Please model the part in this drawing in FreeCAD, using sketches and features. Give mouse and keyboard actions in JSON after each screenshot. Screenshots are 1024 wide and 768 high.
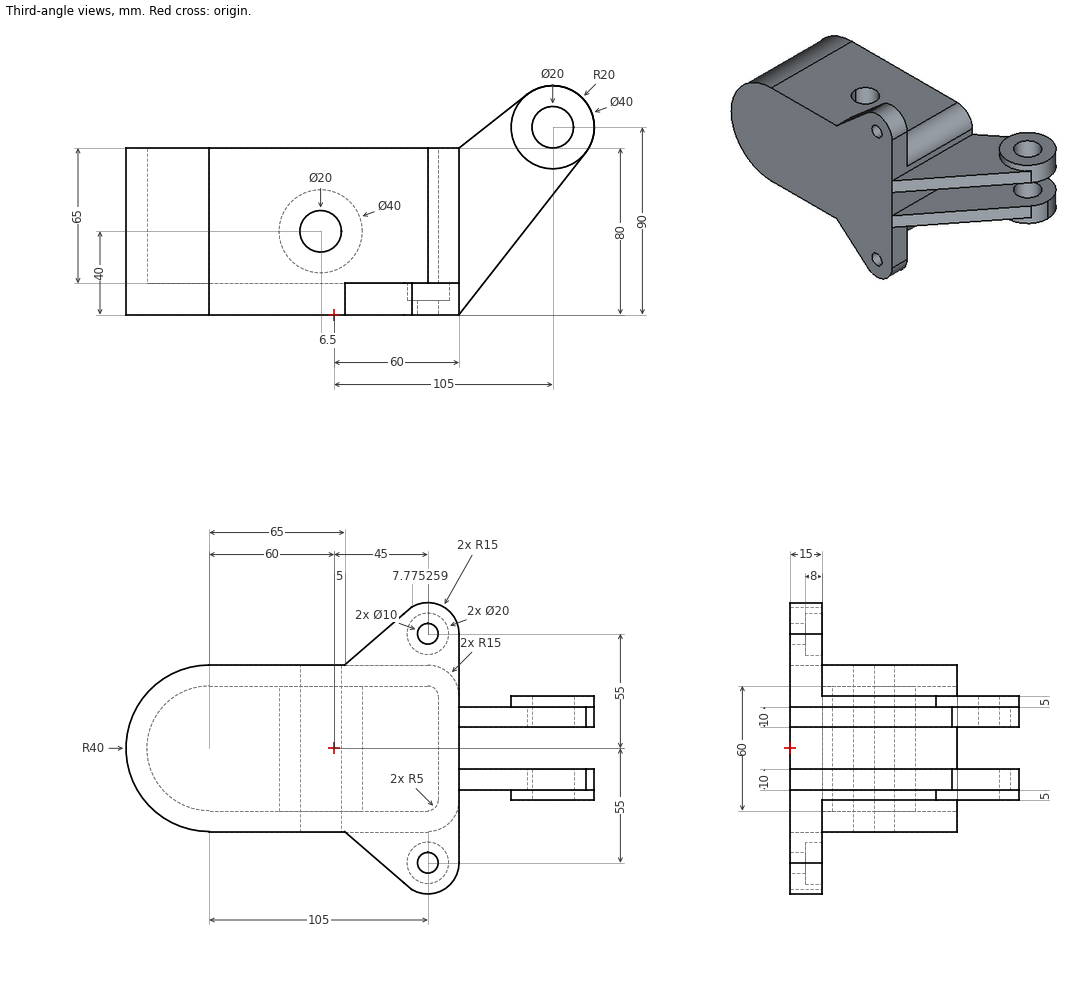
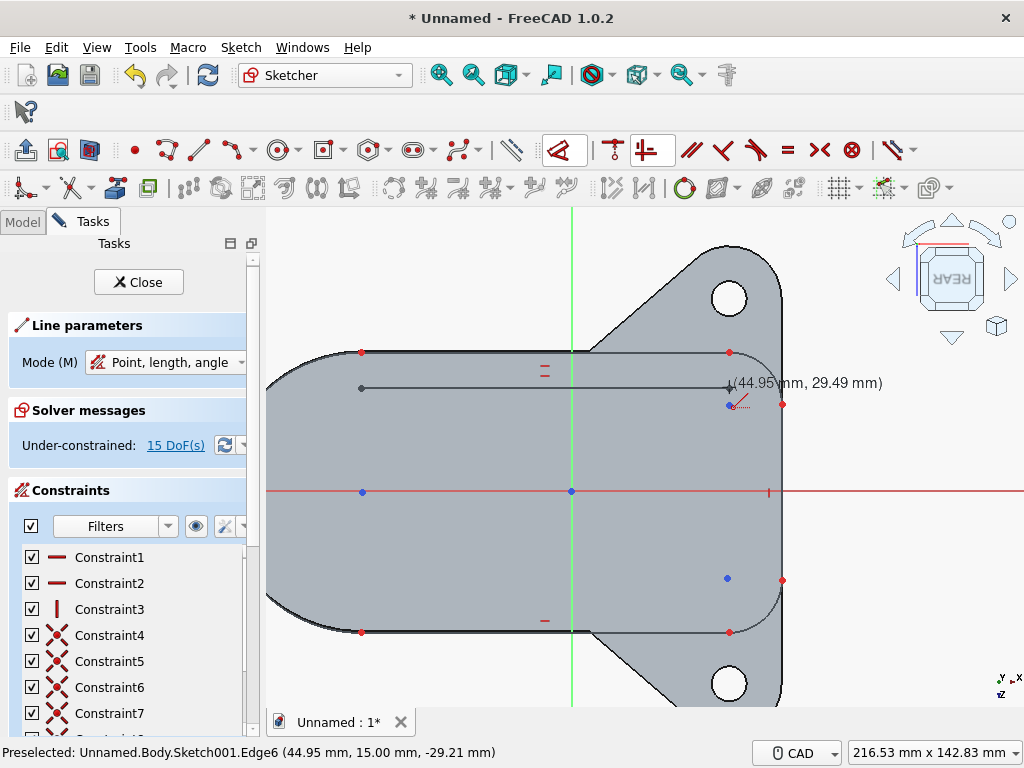
{"action": "left_click", "coordinate": [747, 404]}
{"action": "left_click", "coordinate": [747, 579]}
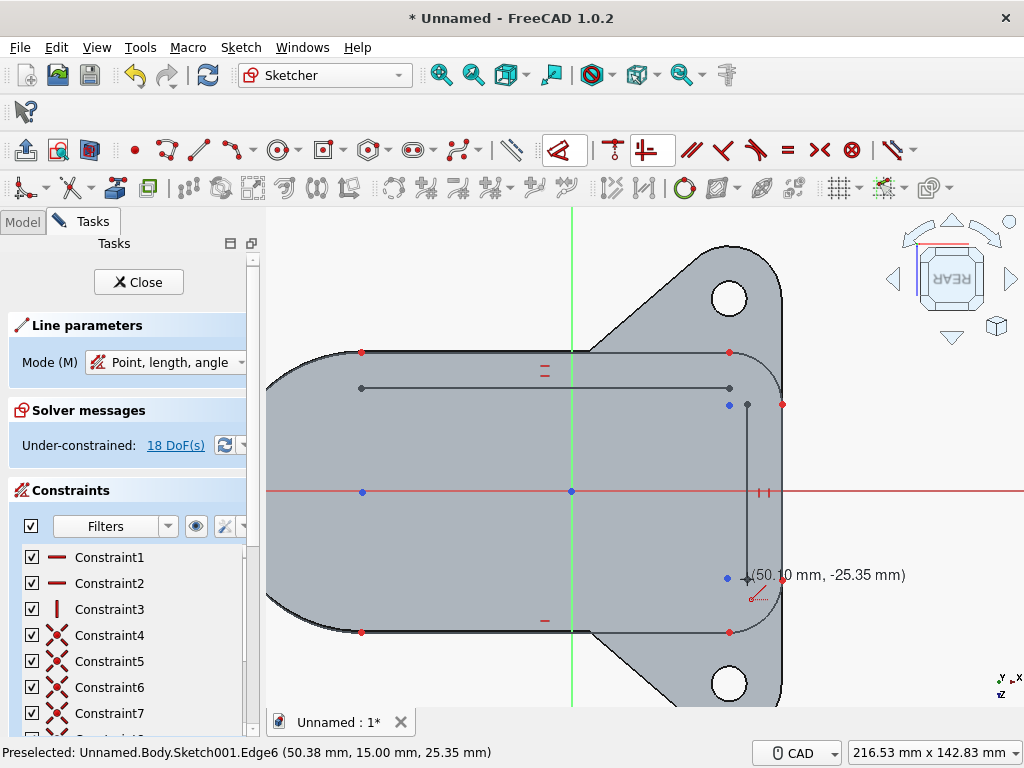
{"action": "left_click", "coordinate": [729, 596]}
{"action": "left_click", "coordinate": [362, 596]}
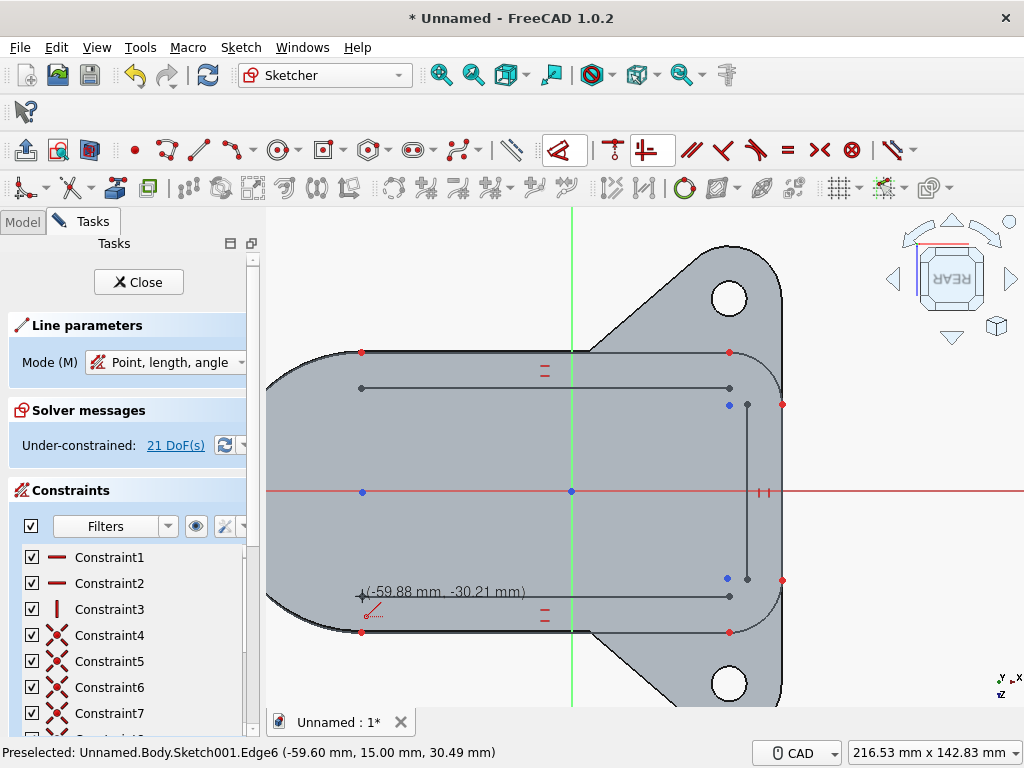
{"action": "left_click", "coordinate": [232, 150]}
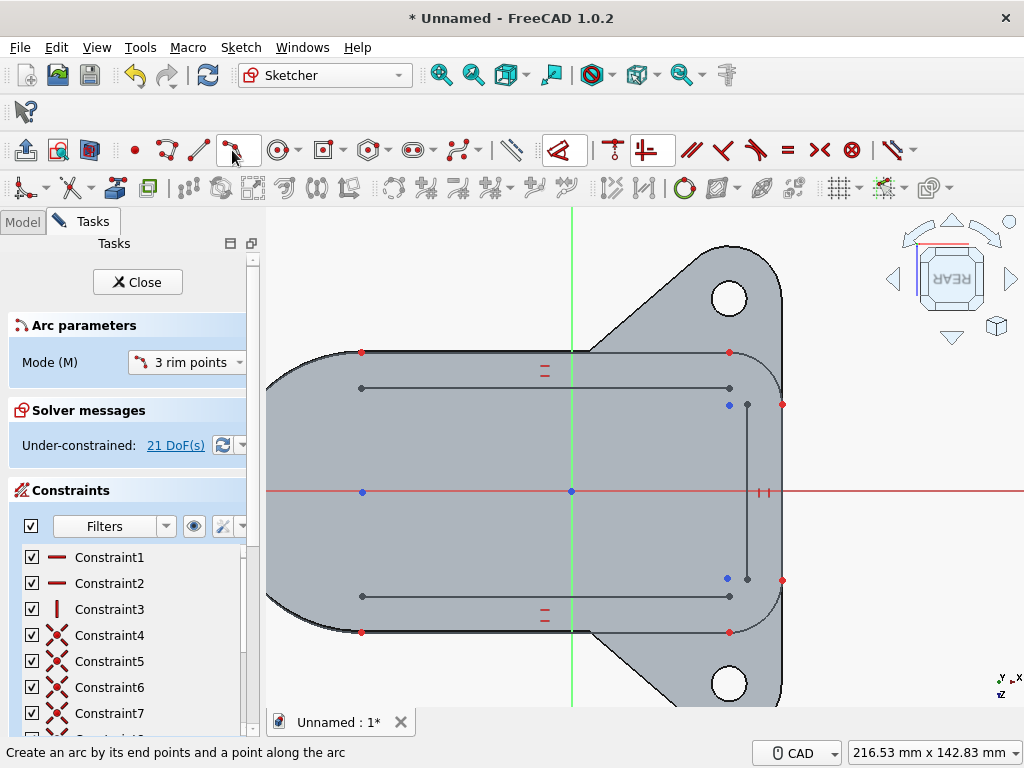
{"action": "left_click", "coordinate": [729, 388]}
{"action": "left_click", "coordinate": [747, 405]}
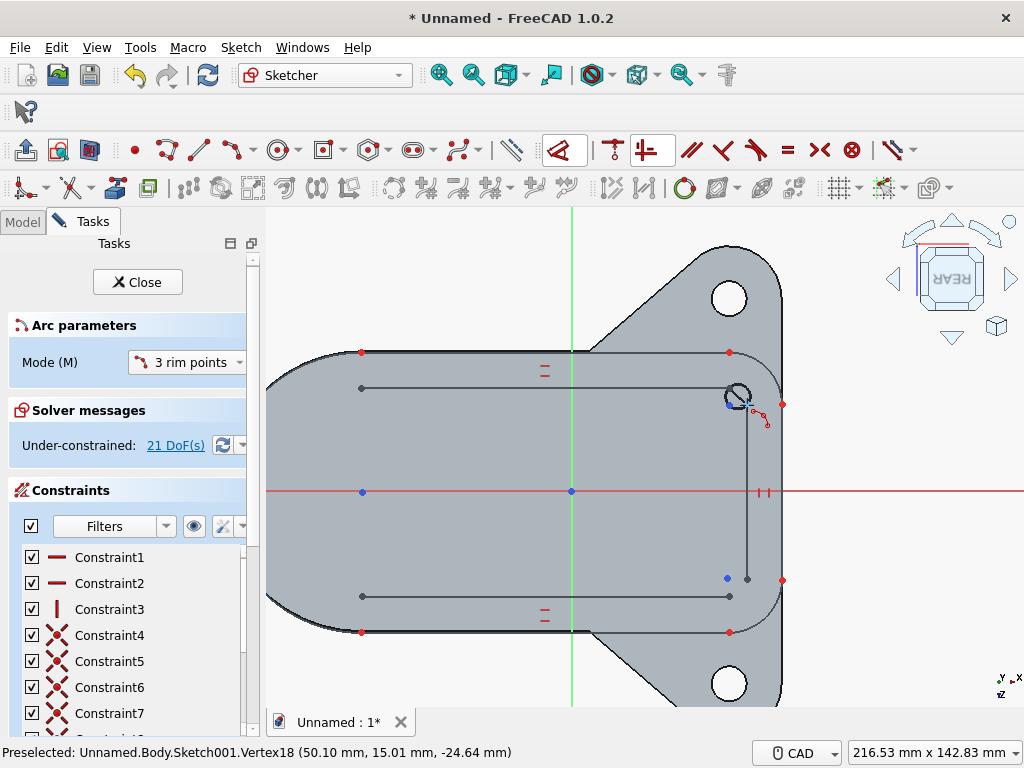
{"action": "scroll", "coordinate": [742, 391], "scroll_direction": "up", "scroll_amount": 6}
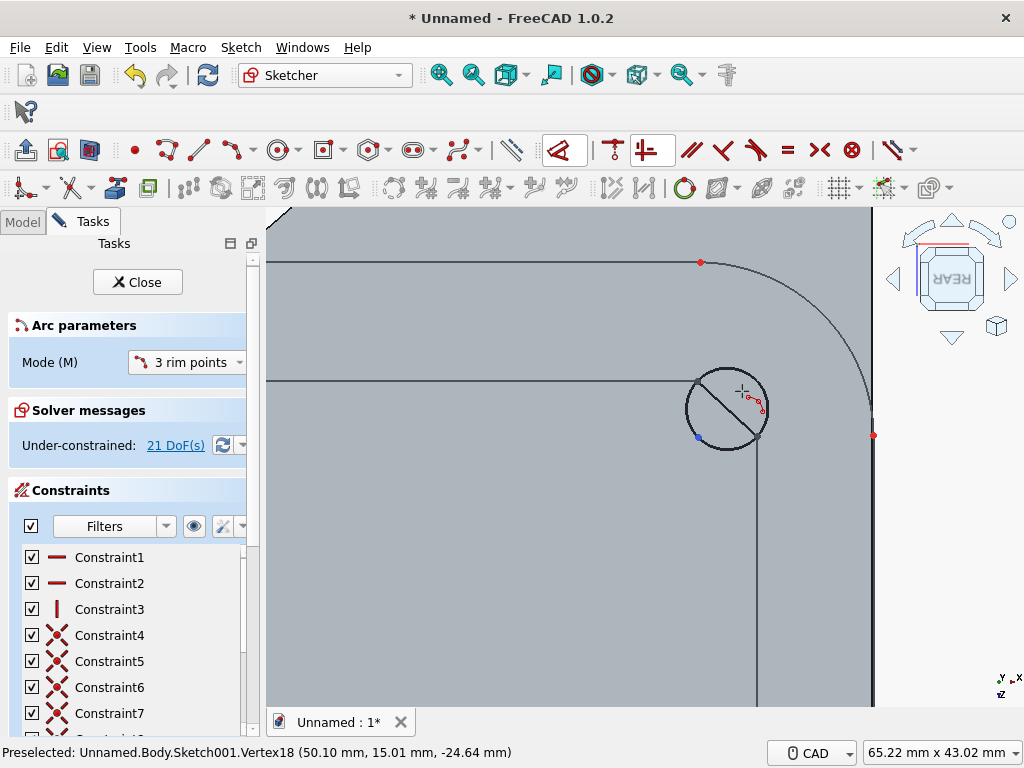
{"action": "left_click", "coordinate": [739, 391]}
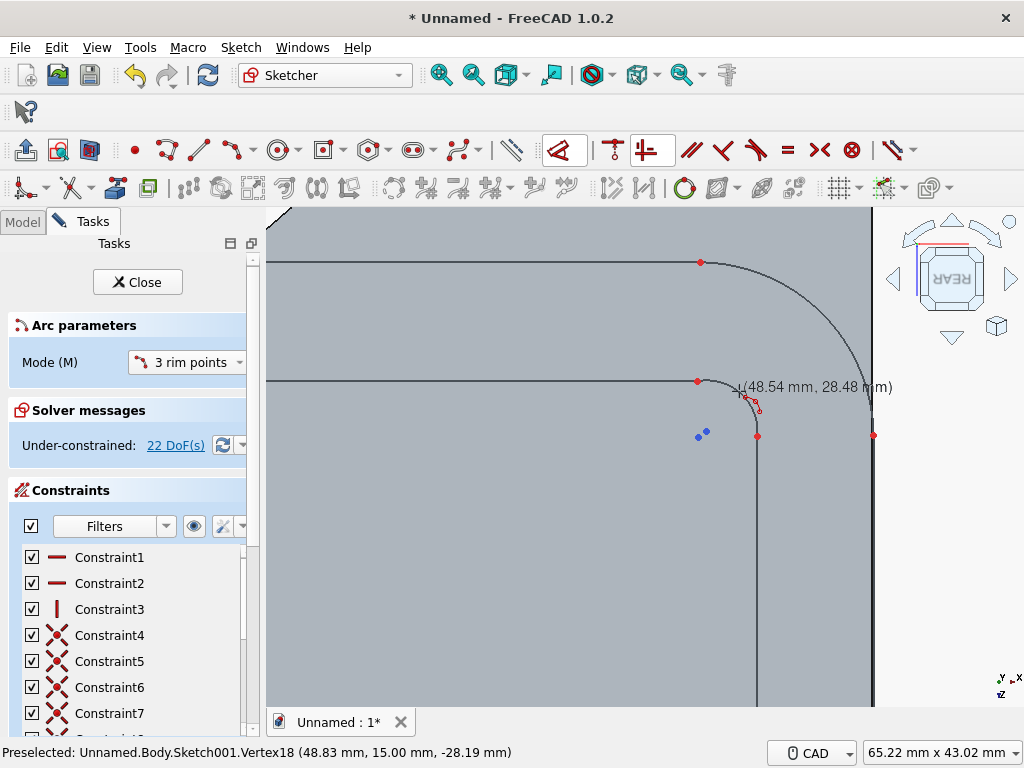
{"action": "scroll", "coordinate": [737, 390], "scroll_direction": "down", "scroll_amount": 8}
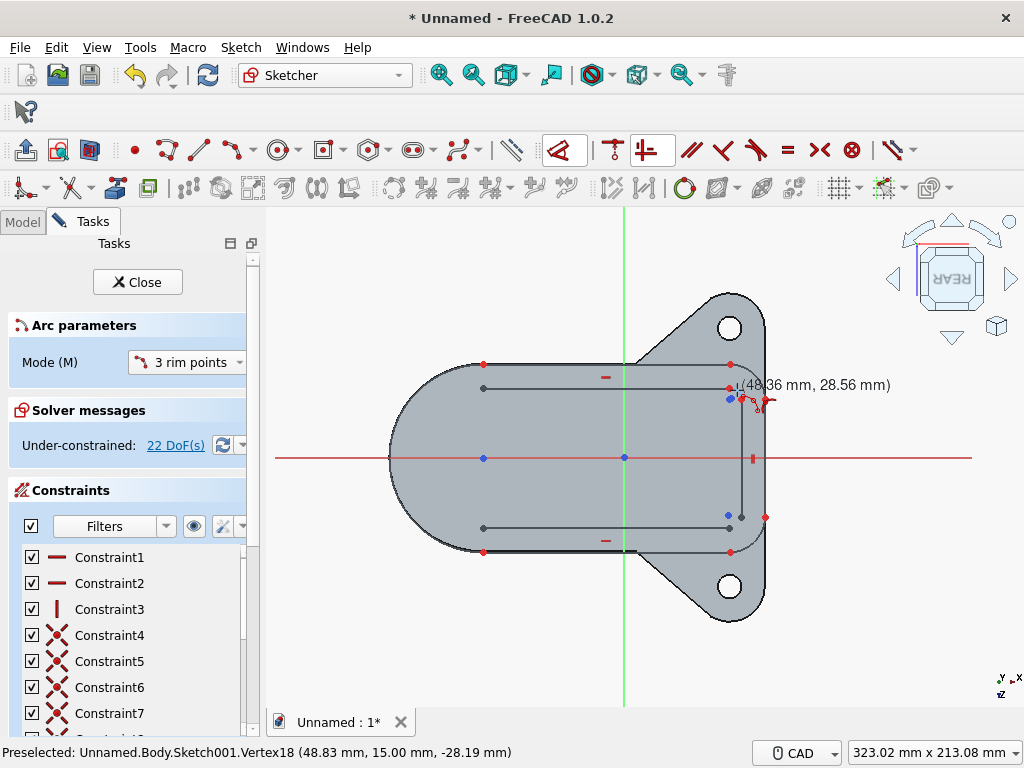
{"action": "scroll", "coordinate": [741, 516], "scroll_direction": "up", "scroll_amount": 2}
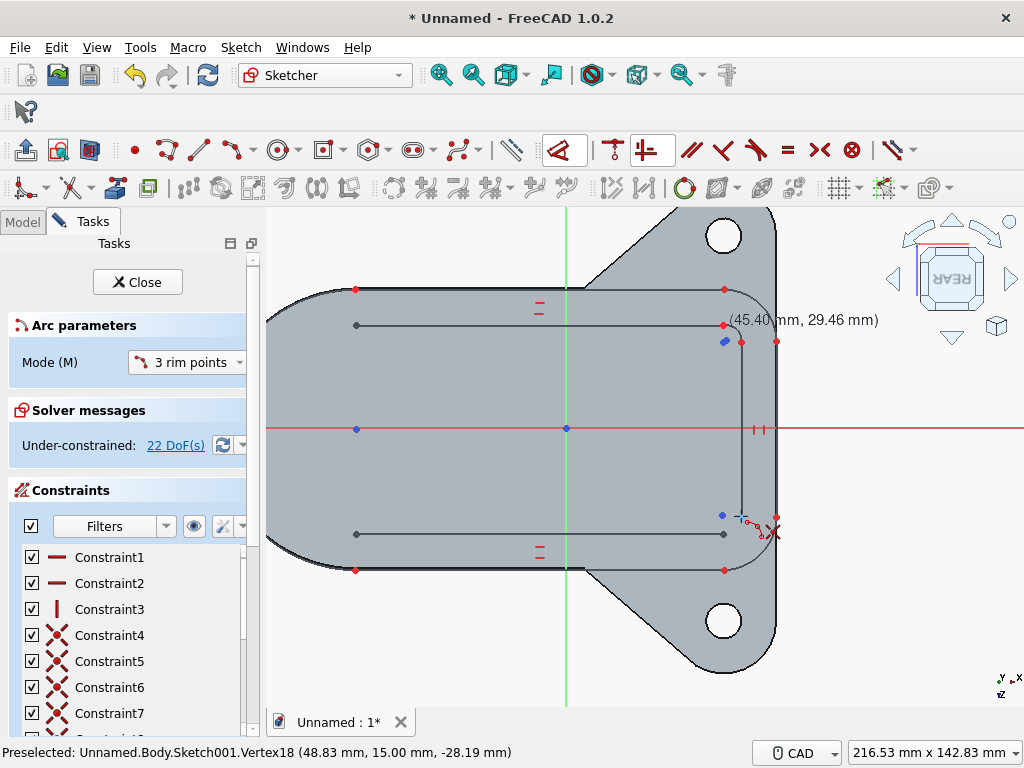
{"action": "left_click", "coordinate": [742, 517]}
{"action": "left_click", "coordinate": [724, 534]}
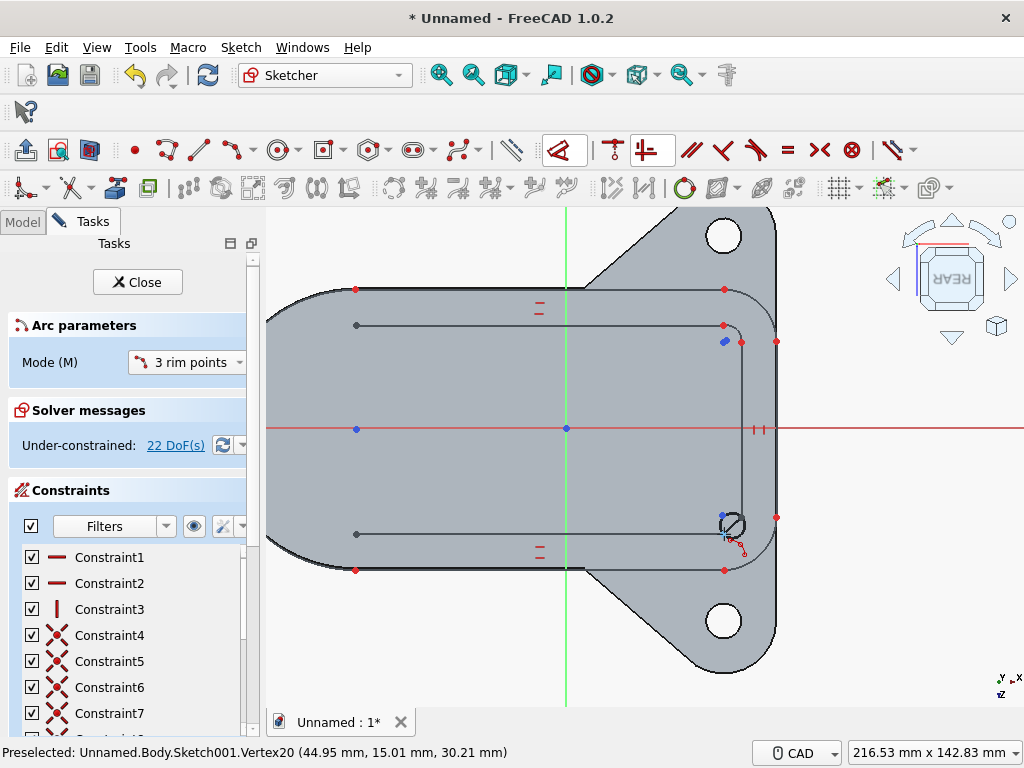
{"action": "scroll", "coordinate": [736, 528], "scroll_direction": "up", "scroll_amount": 6}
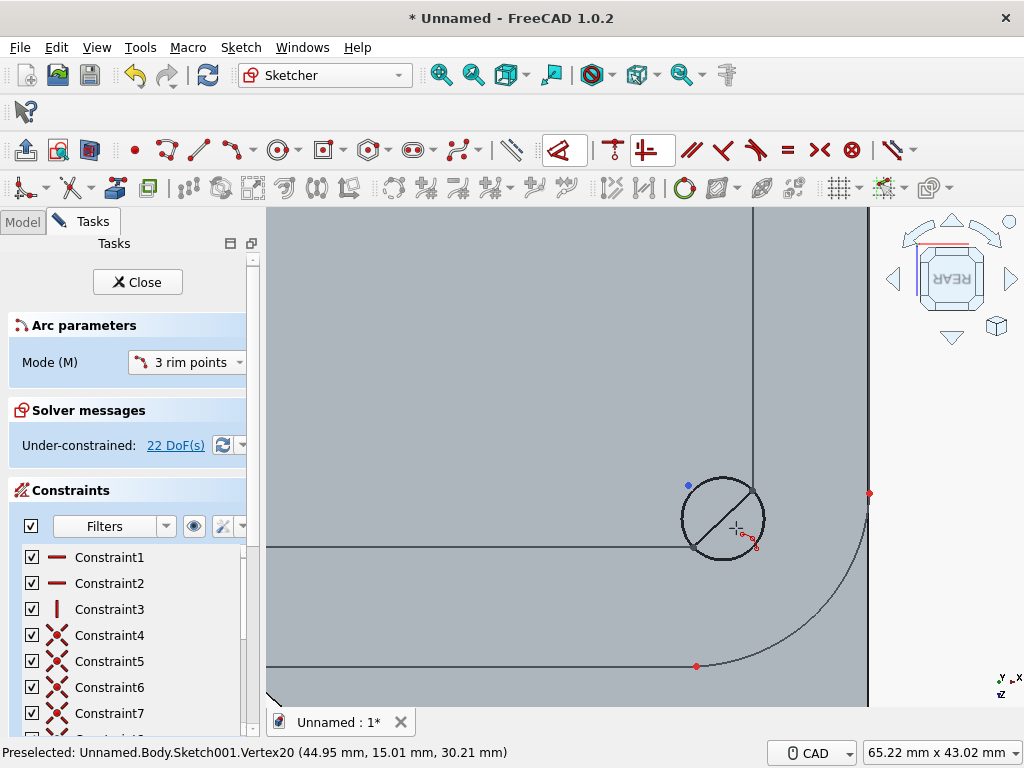
{"action": "left_click", "coordinate": [735, 528]}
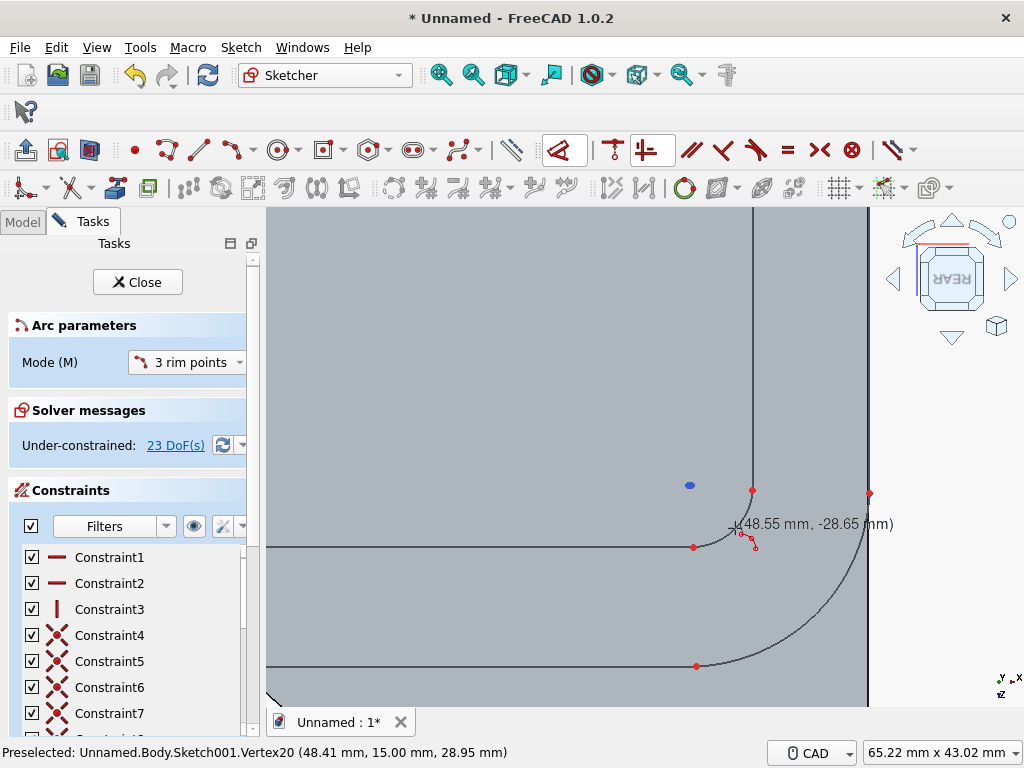
{"action": "scroll", "coordinate": [738, 523], "scroll_direction": "down", "scroll_amount": 8}